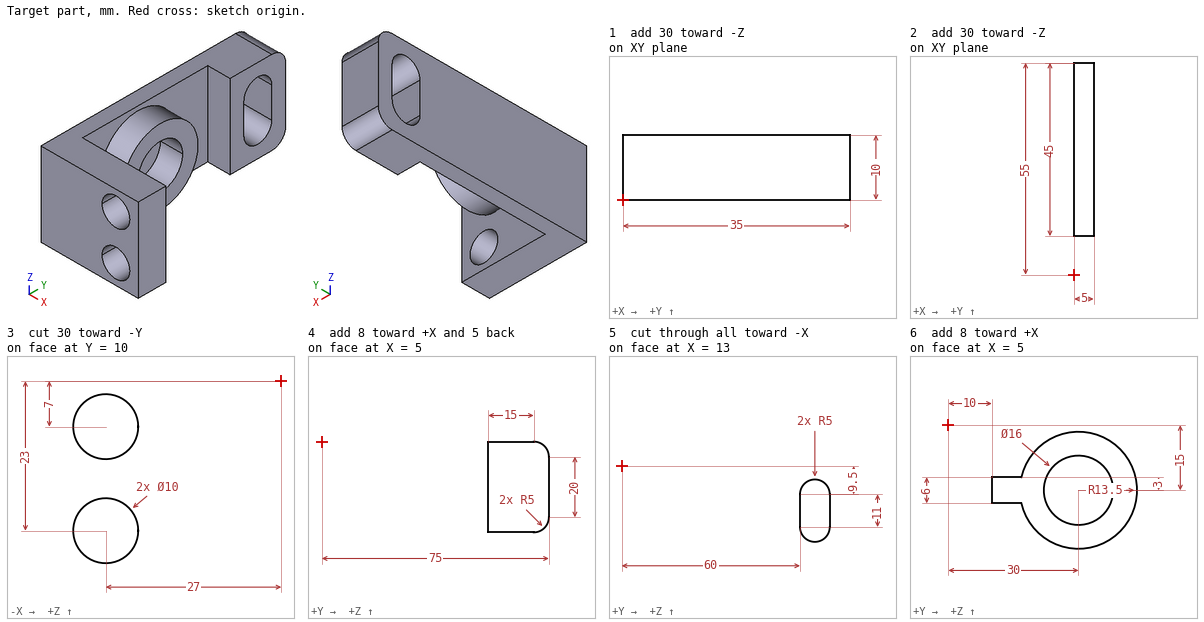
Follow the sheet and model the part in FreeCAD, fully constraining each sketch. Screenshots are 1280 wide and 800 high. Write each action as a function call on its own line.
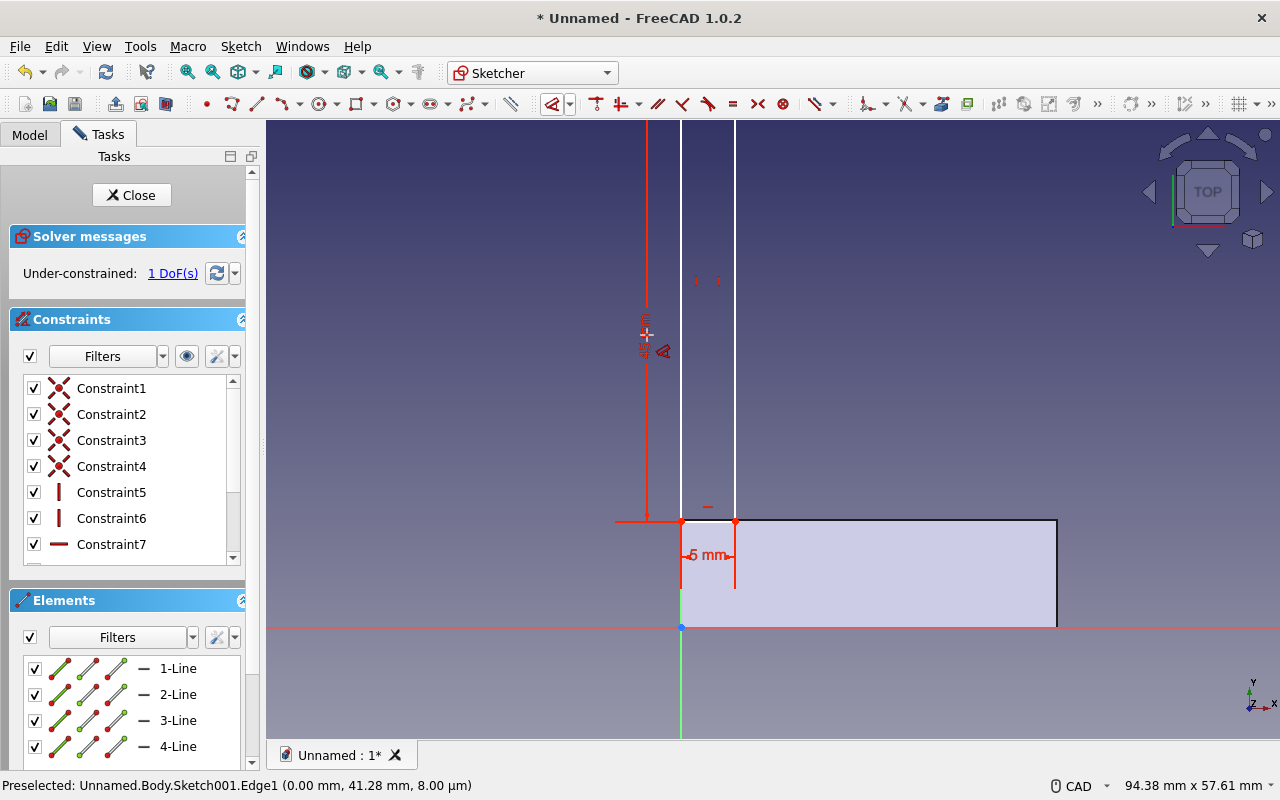
scroll(697, 628, down, 2)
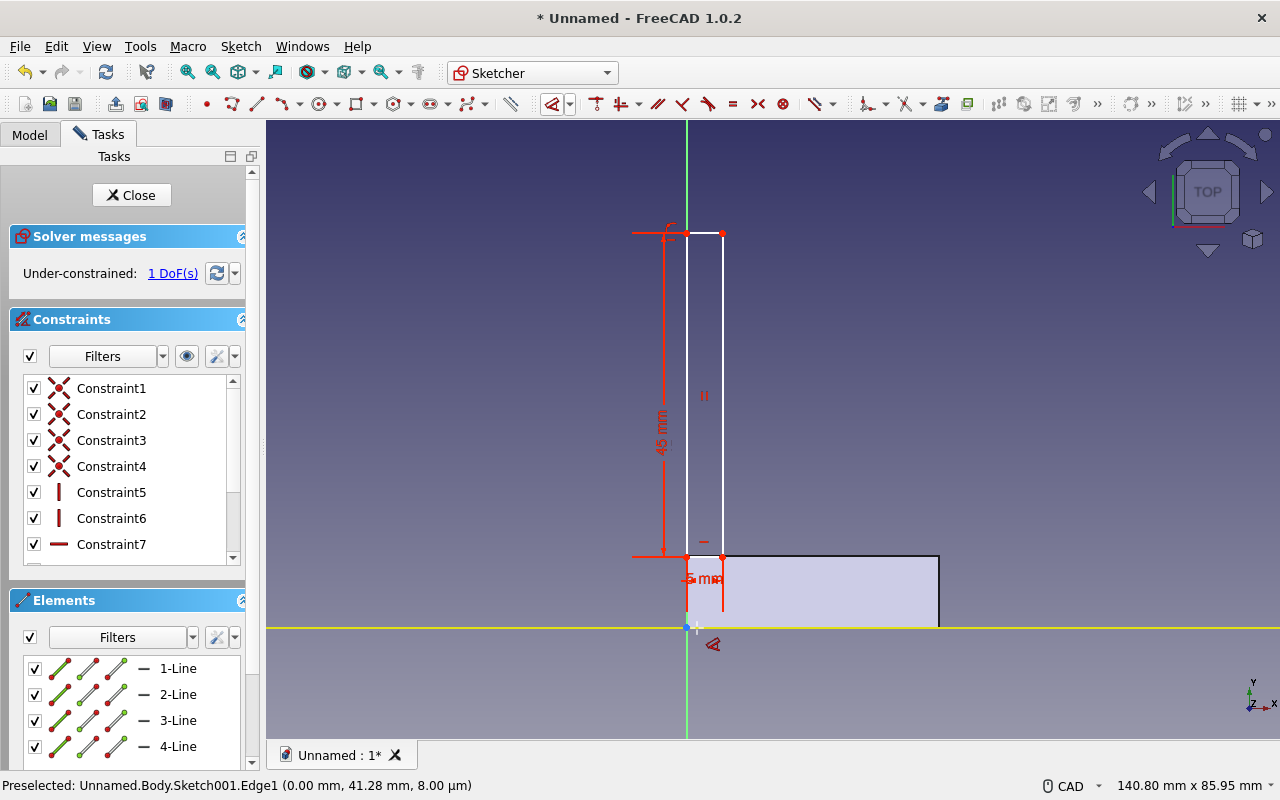
click(687, 233)
click(653, 340)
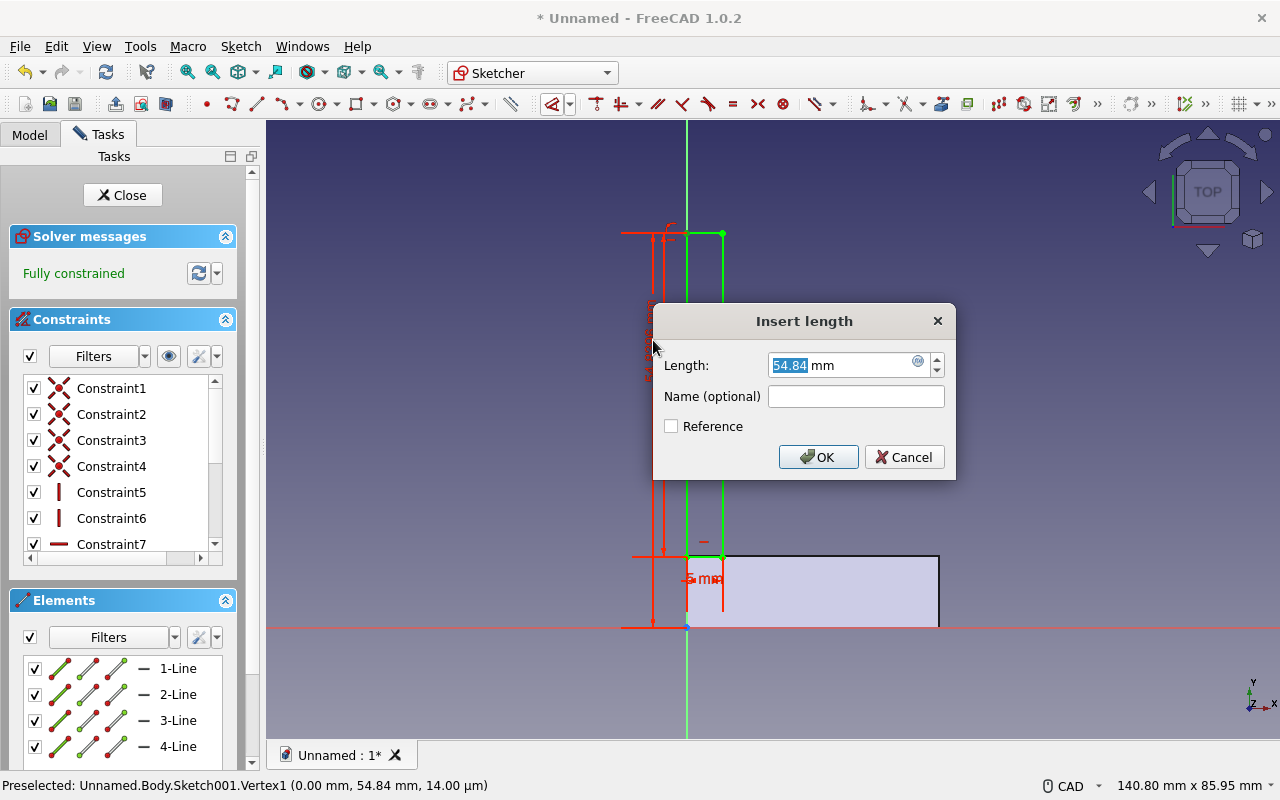
text(55)
key(Return)
key(Escape)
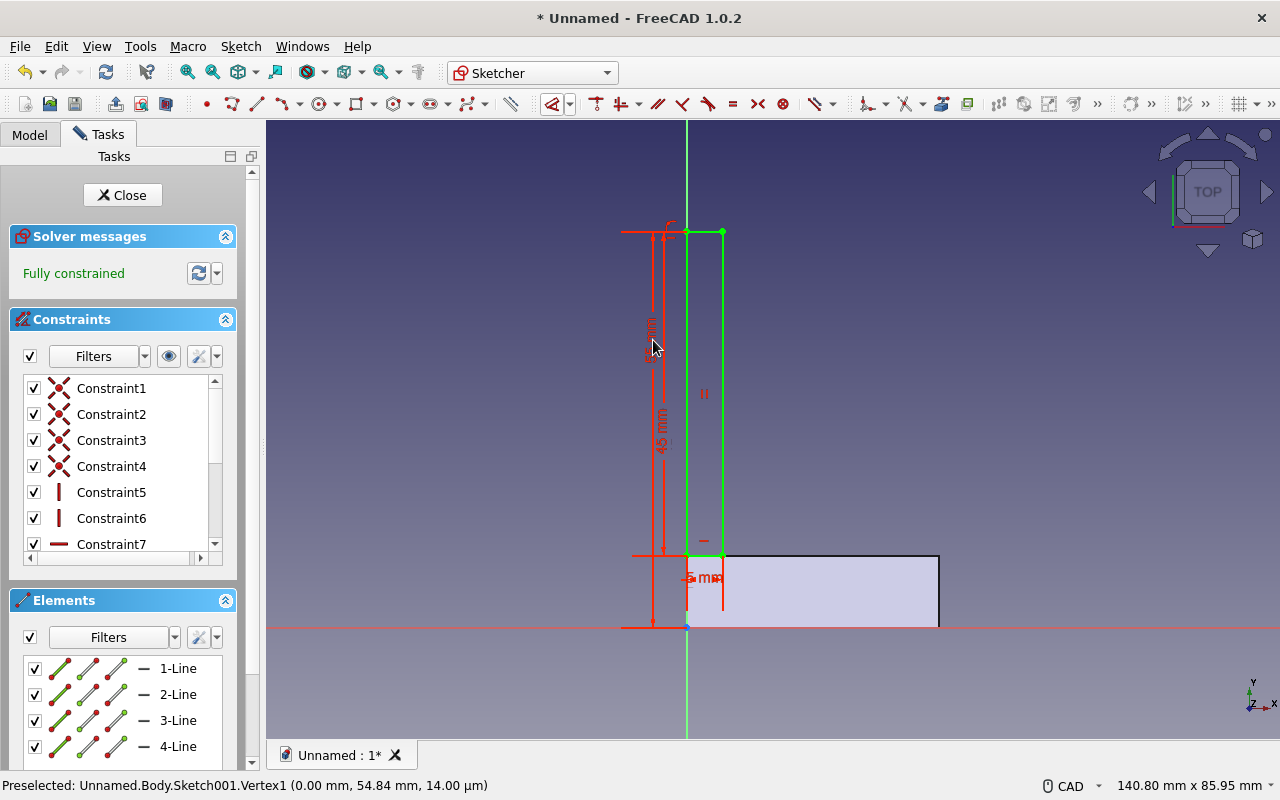
click(123, 195)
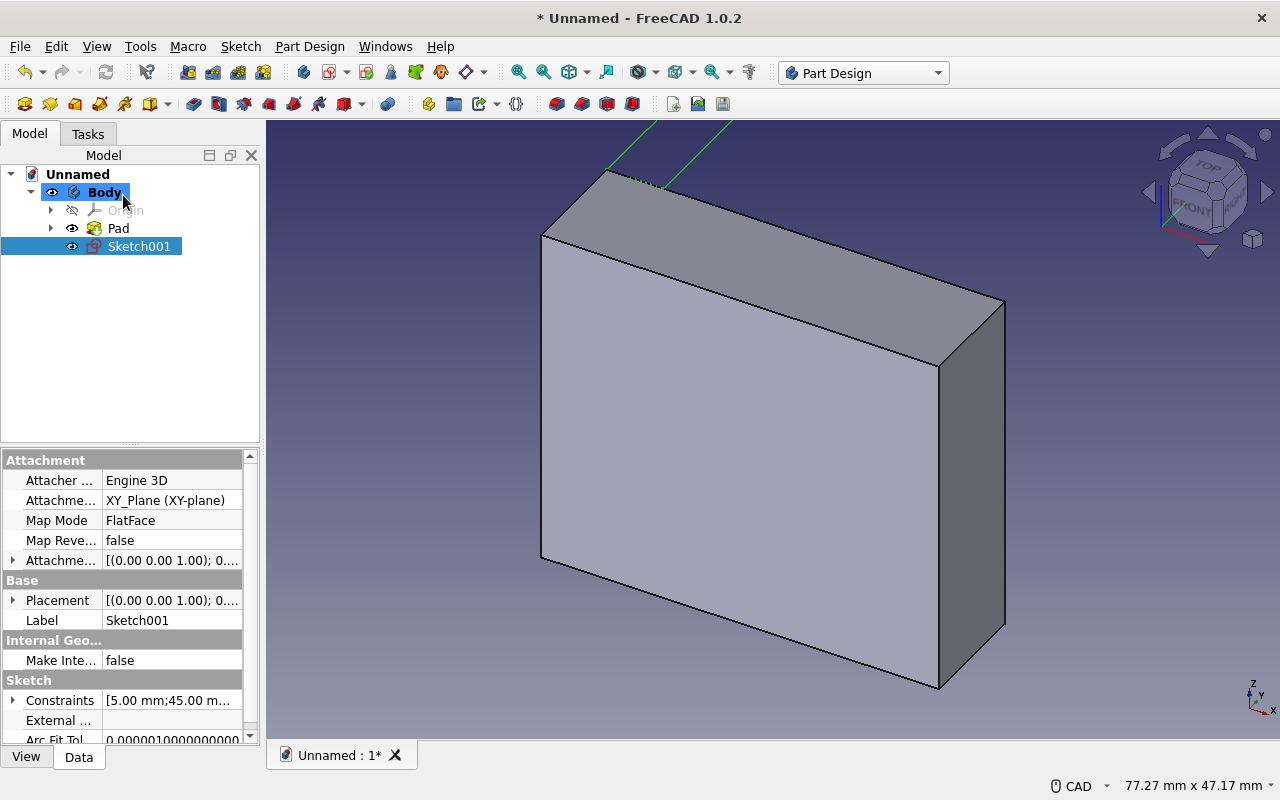
click(25, 104)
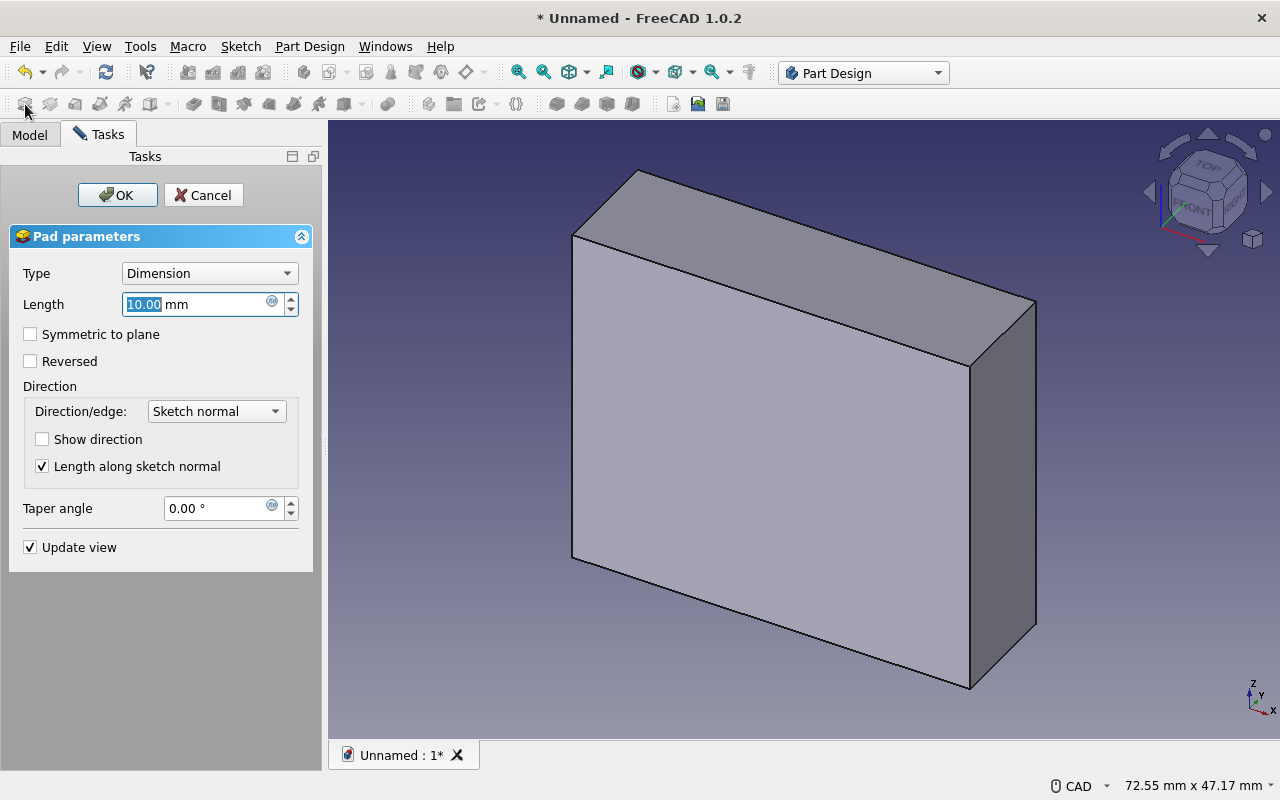
text(30)
key(Tab)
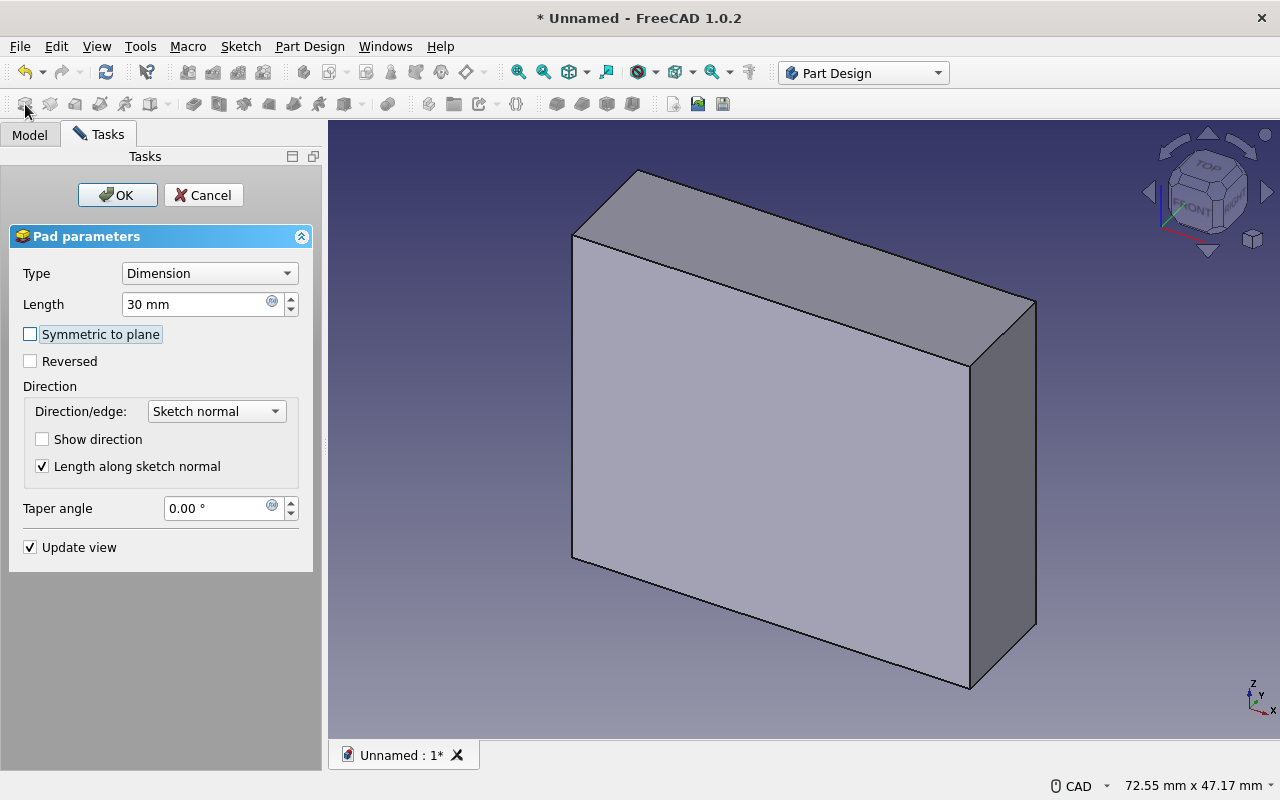
click(31, 361)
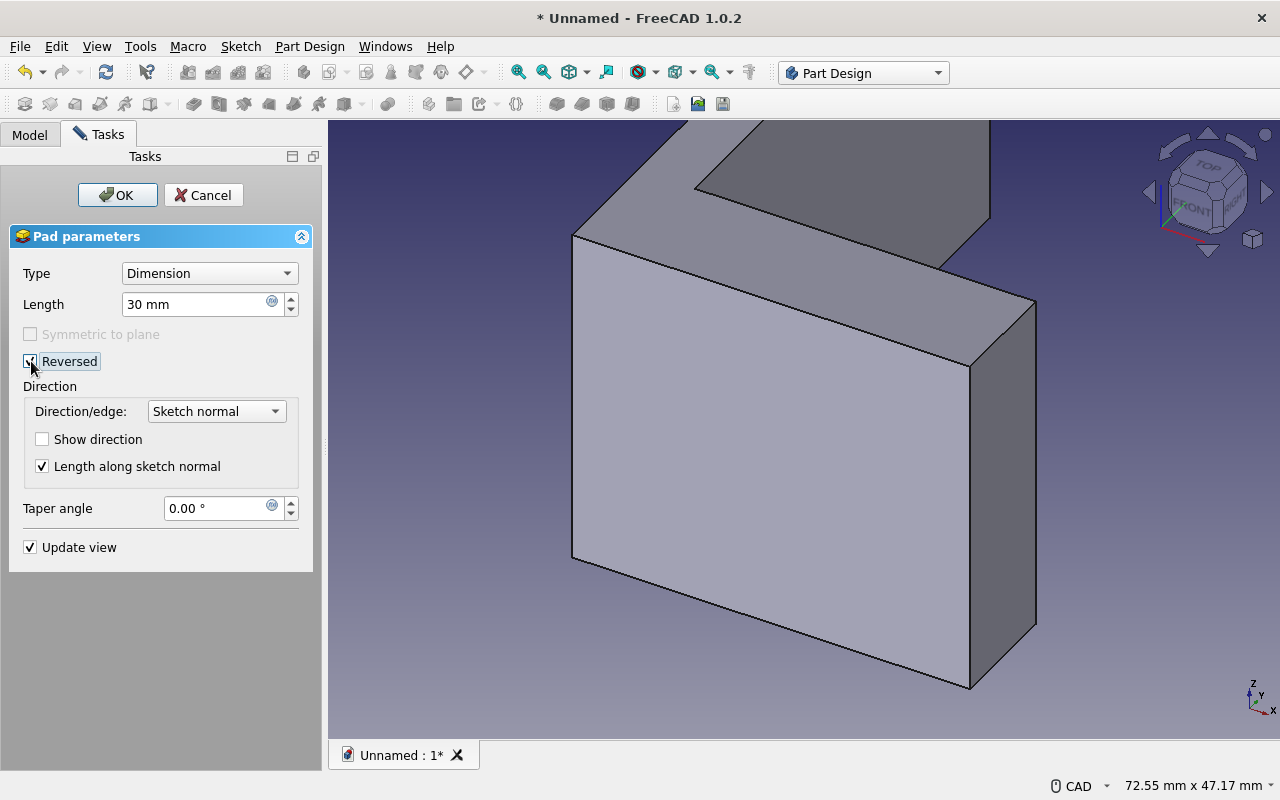
click(118, 195)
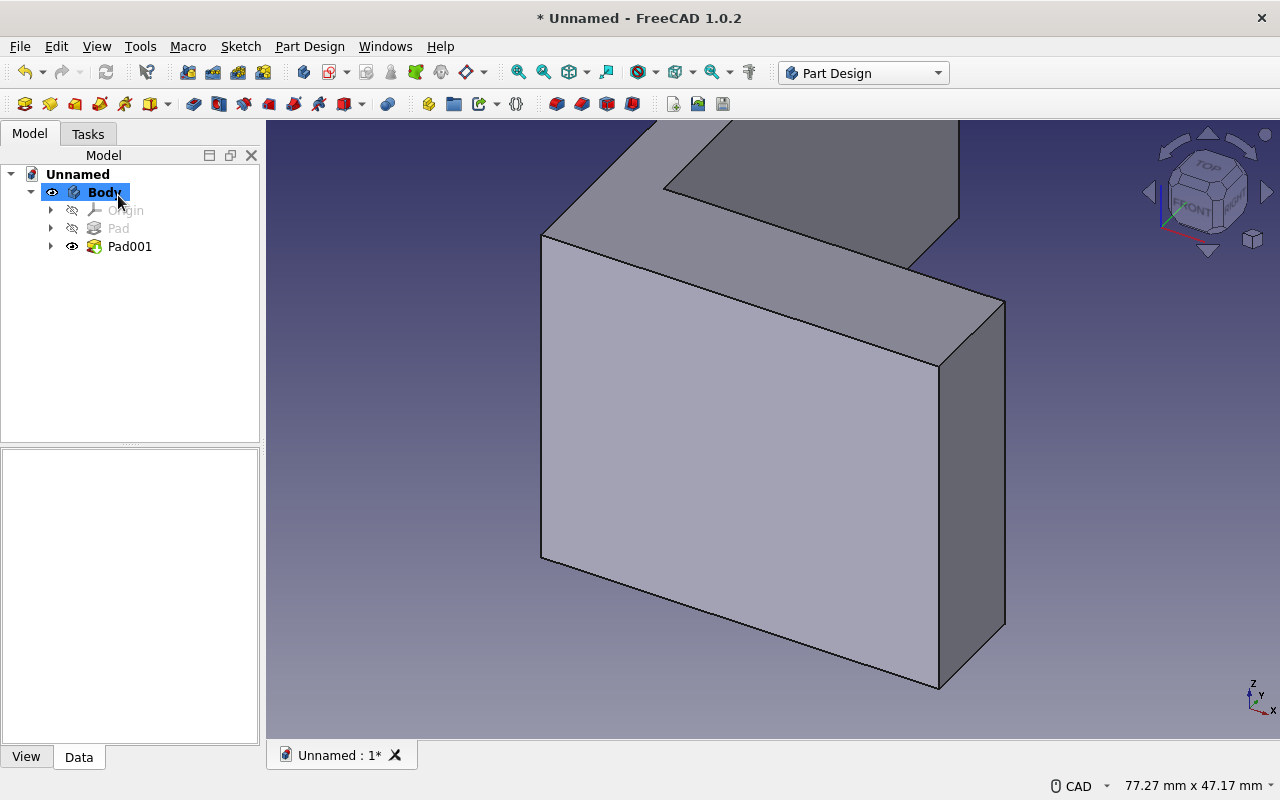
click(519, 72)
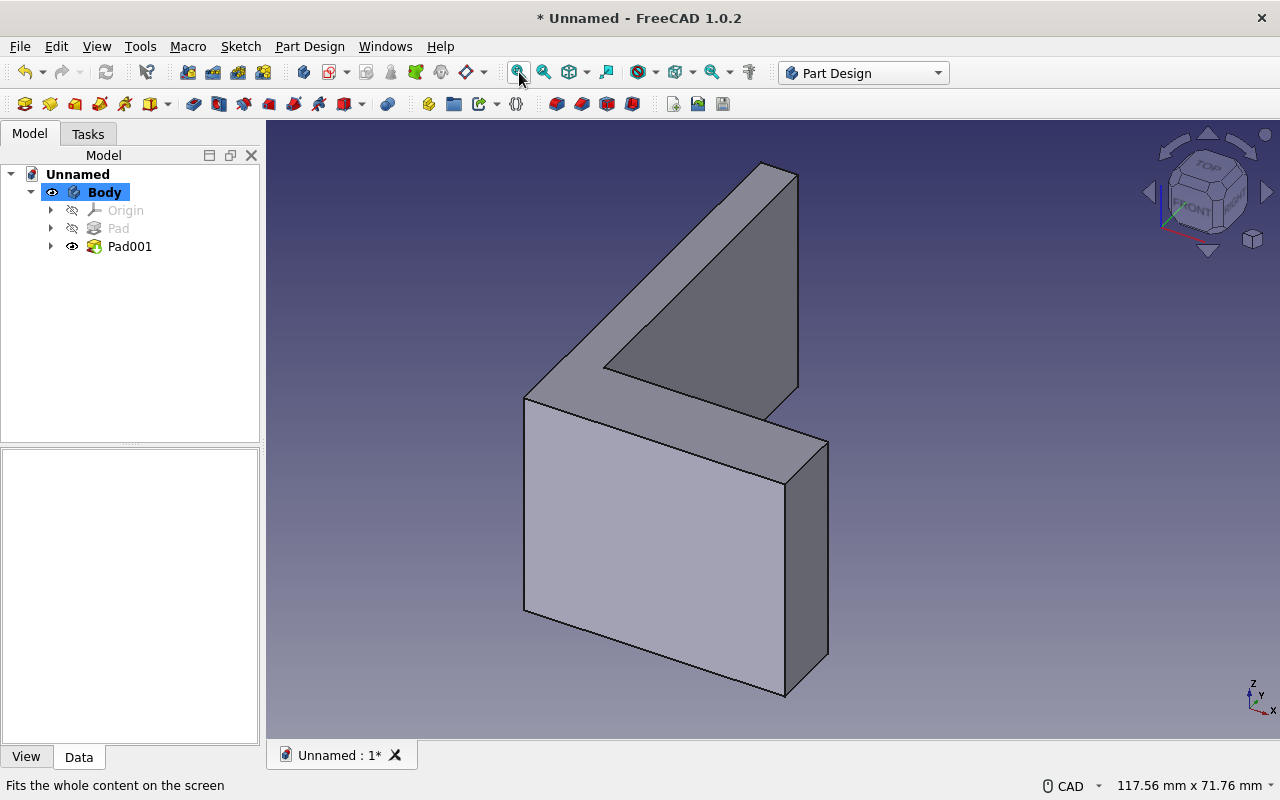
key(4)